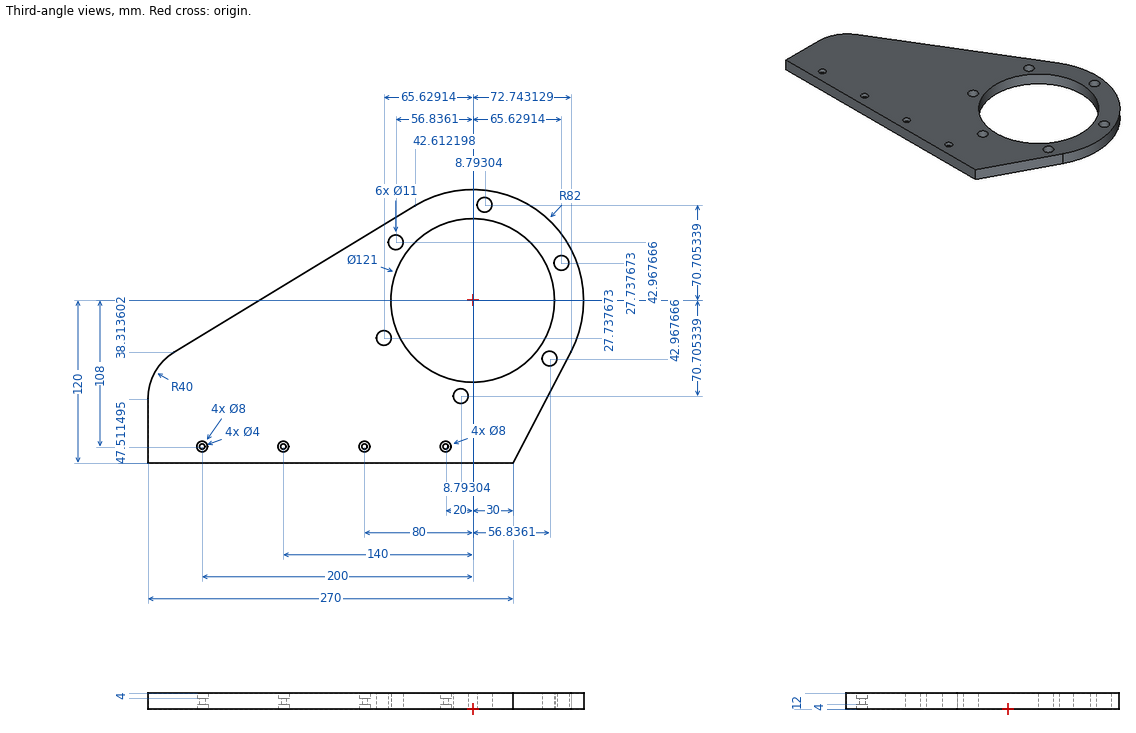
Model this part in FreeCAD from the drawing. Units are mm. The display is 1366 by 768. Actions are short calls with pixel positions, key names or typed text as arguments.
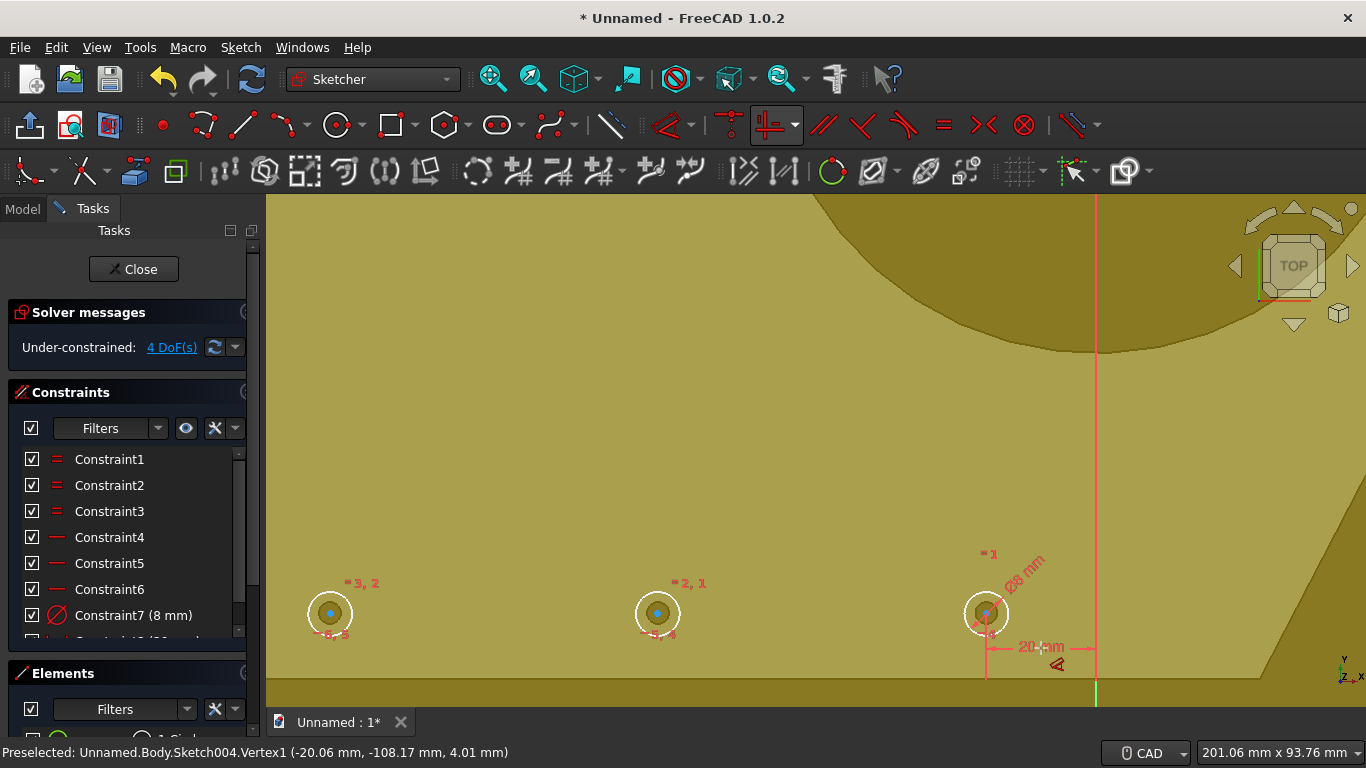
click(658, 614)
click(877, 648)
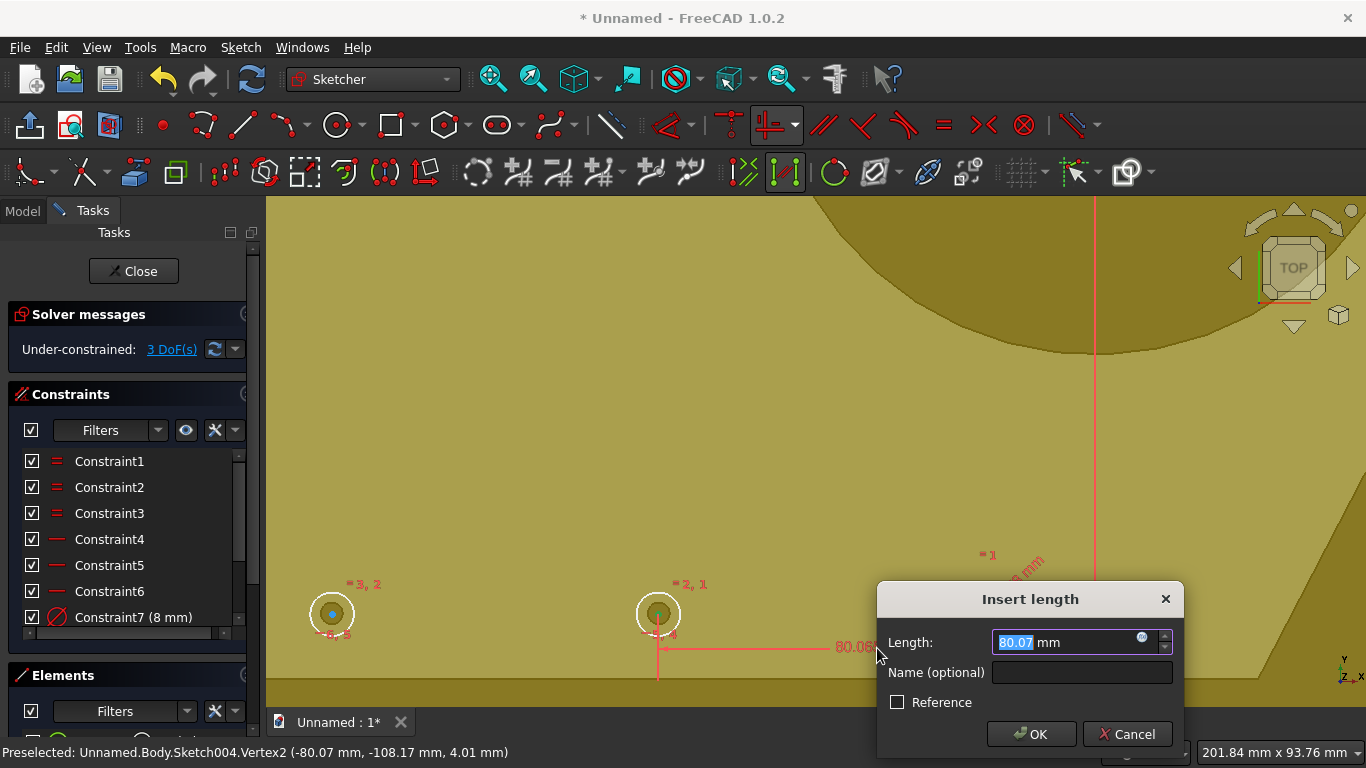
text(80)
key(Return)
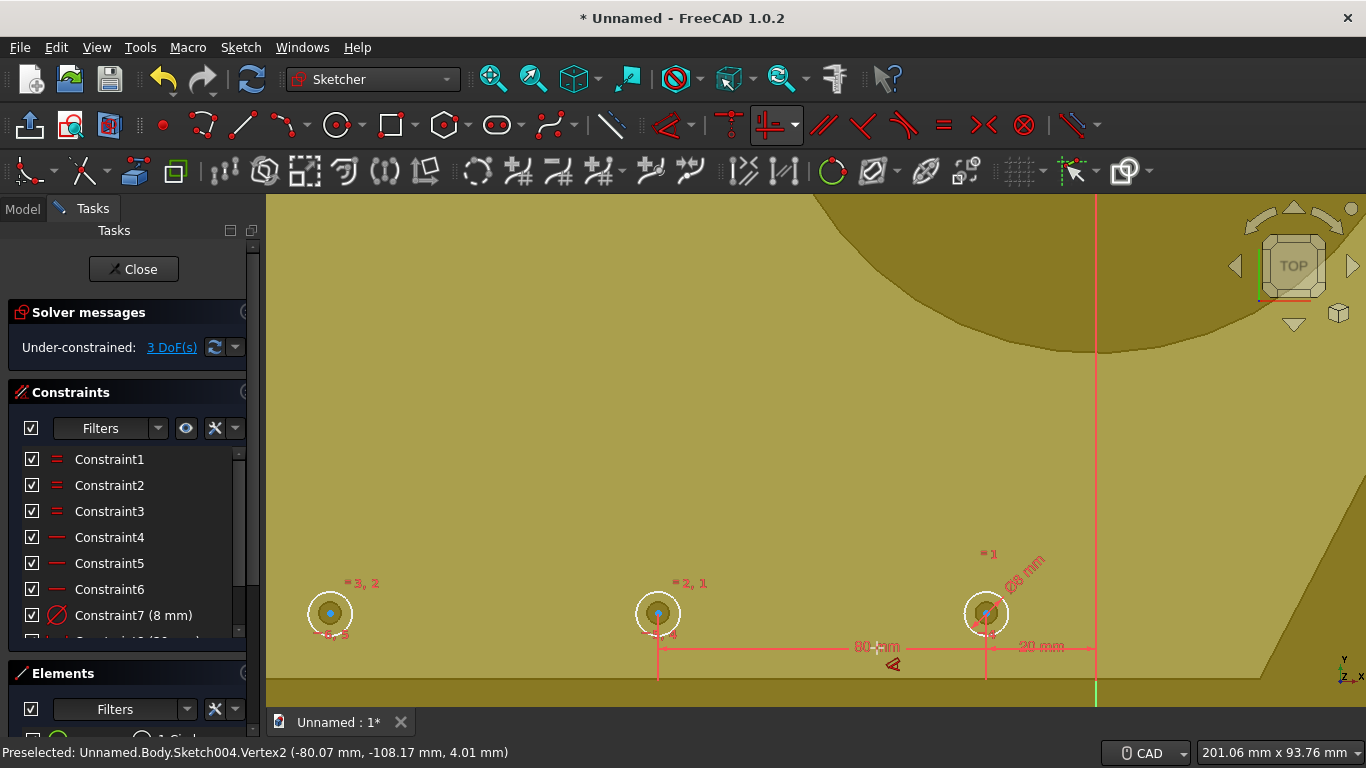
click(986, 614)
click(1130, 418)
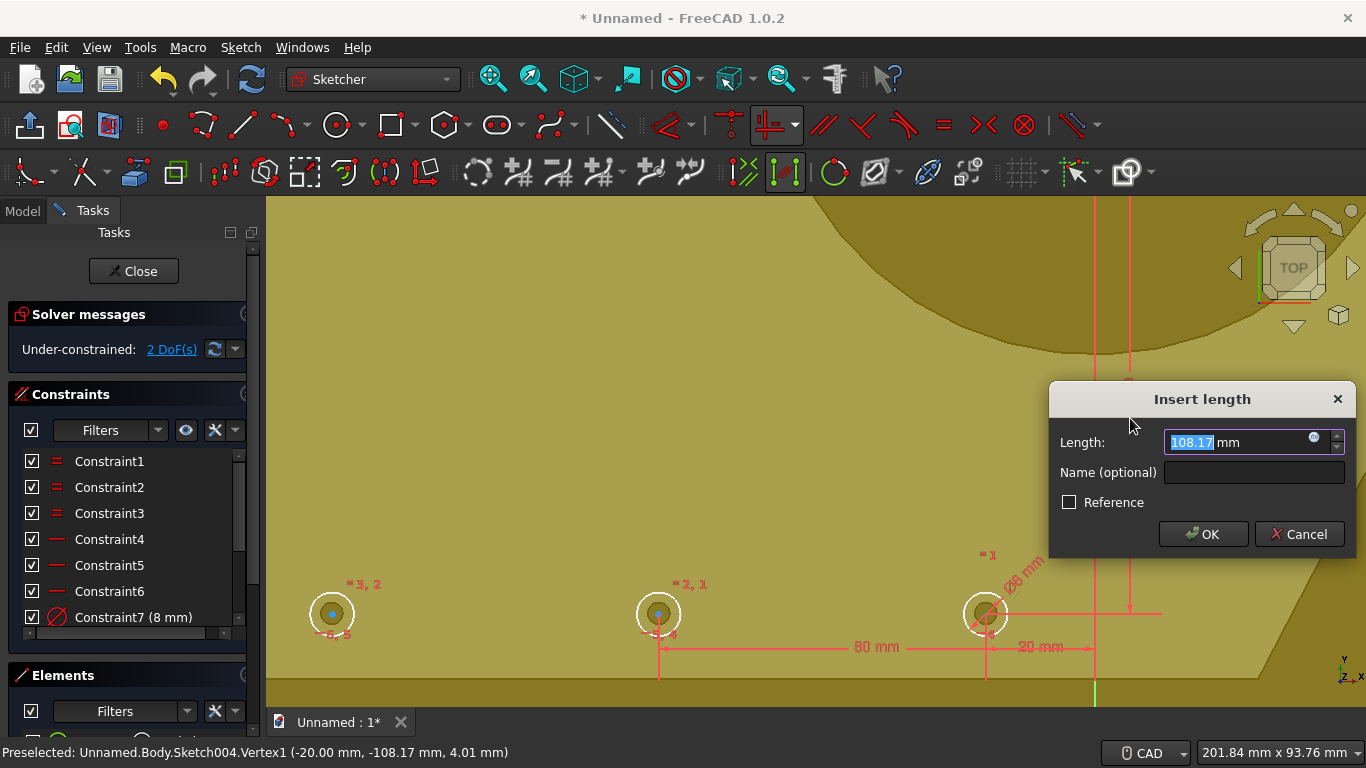
text(108)
key(Return)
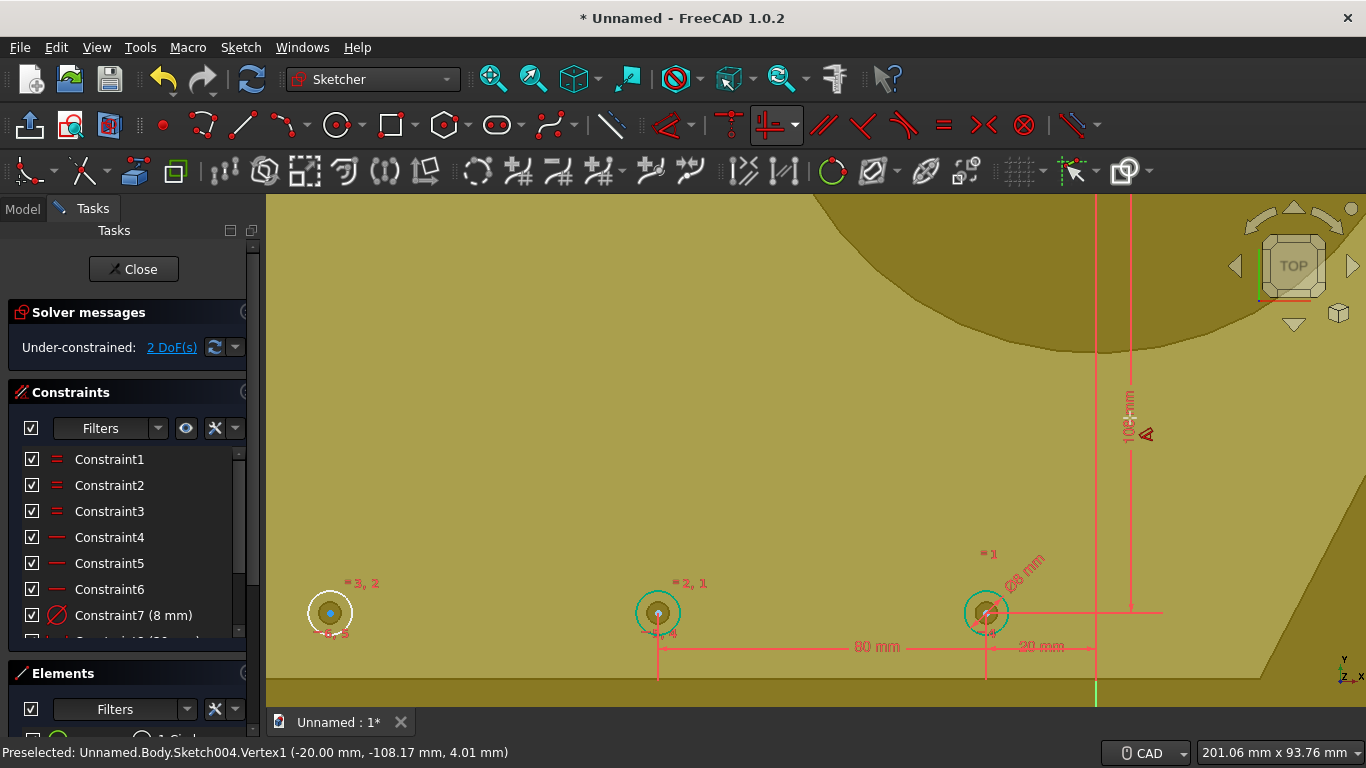
click(330, 613)
click(713, 647)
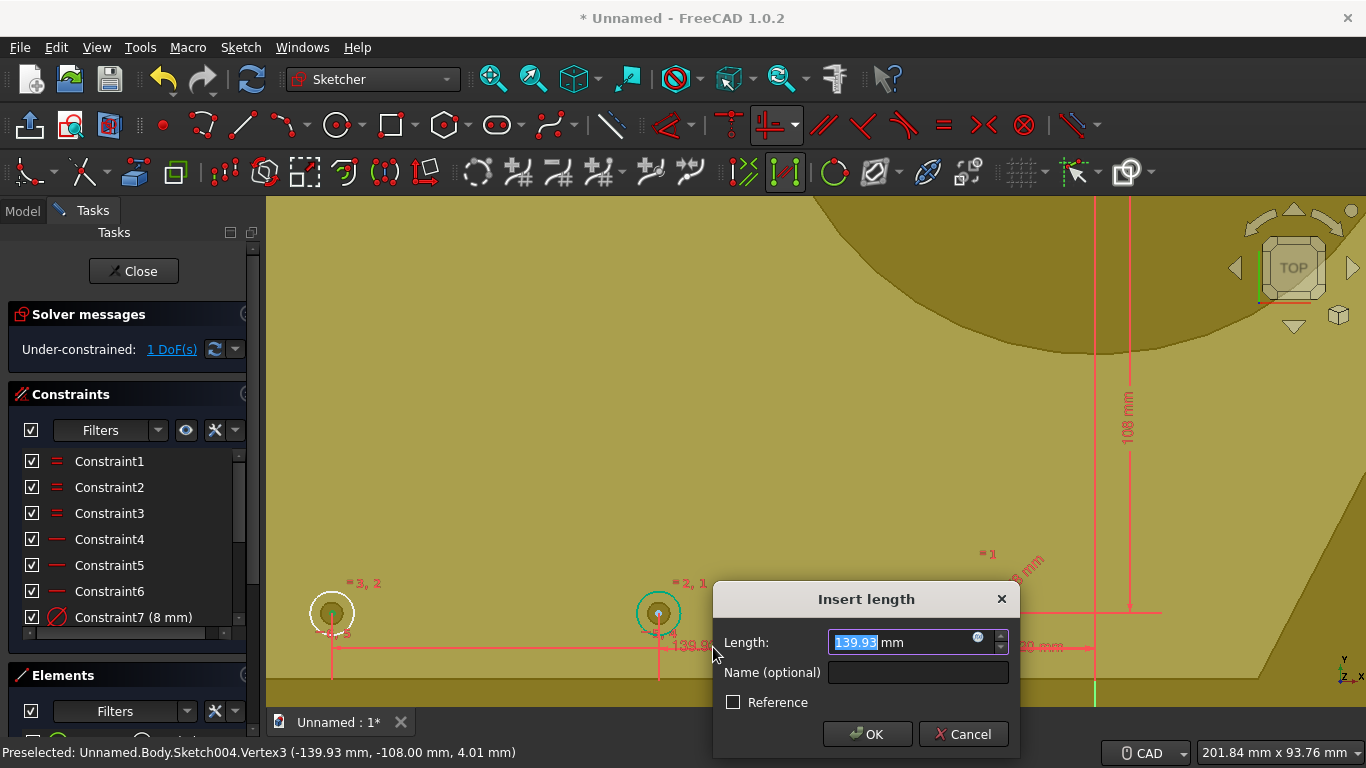
text(140)
key(Return)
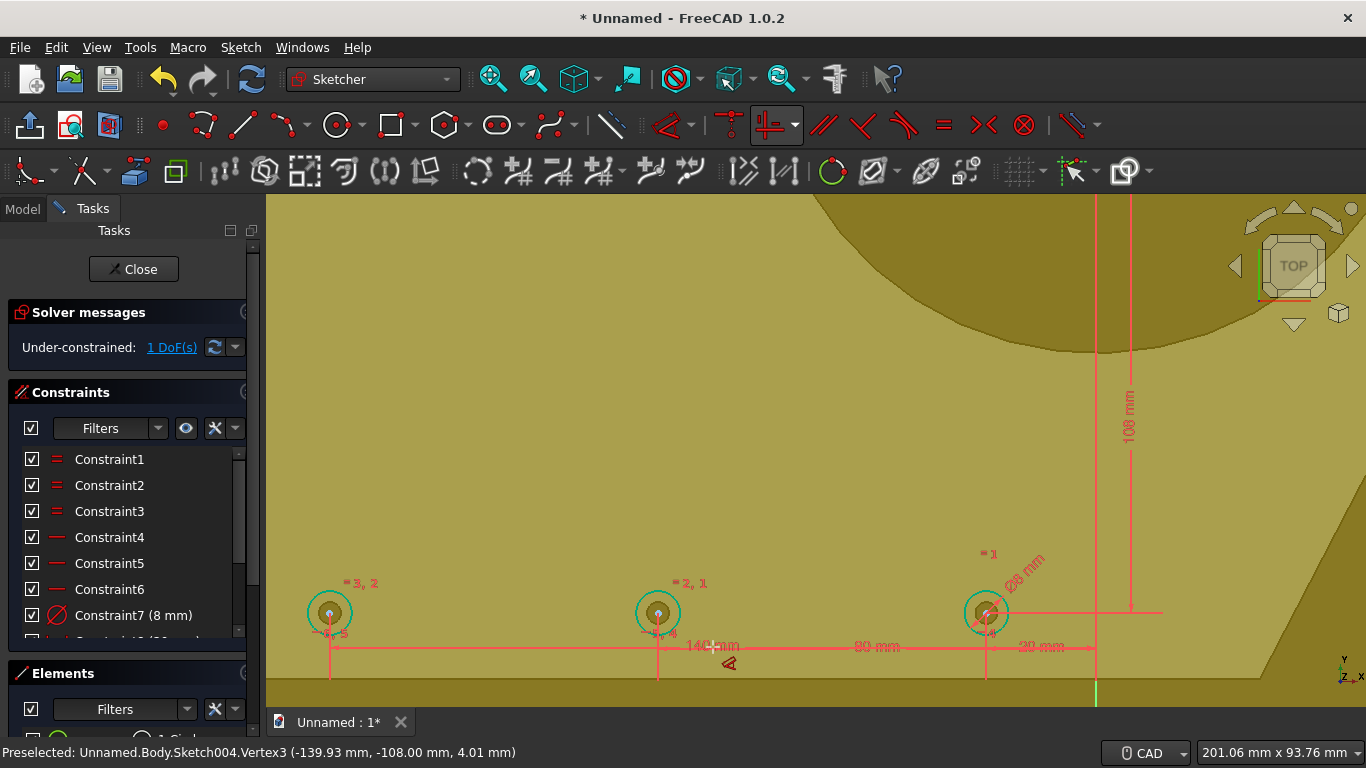
scroll(1003, 599, down, 3)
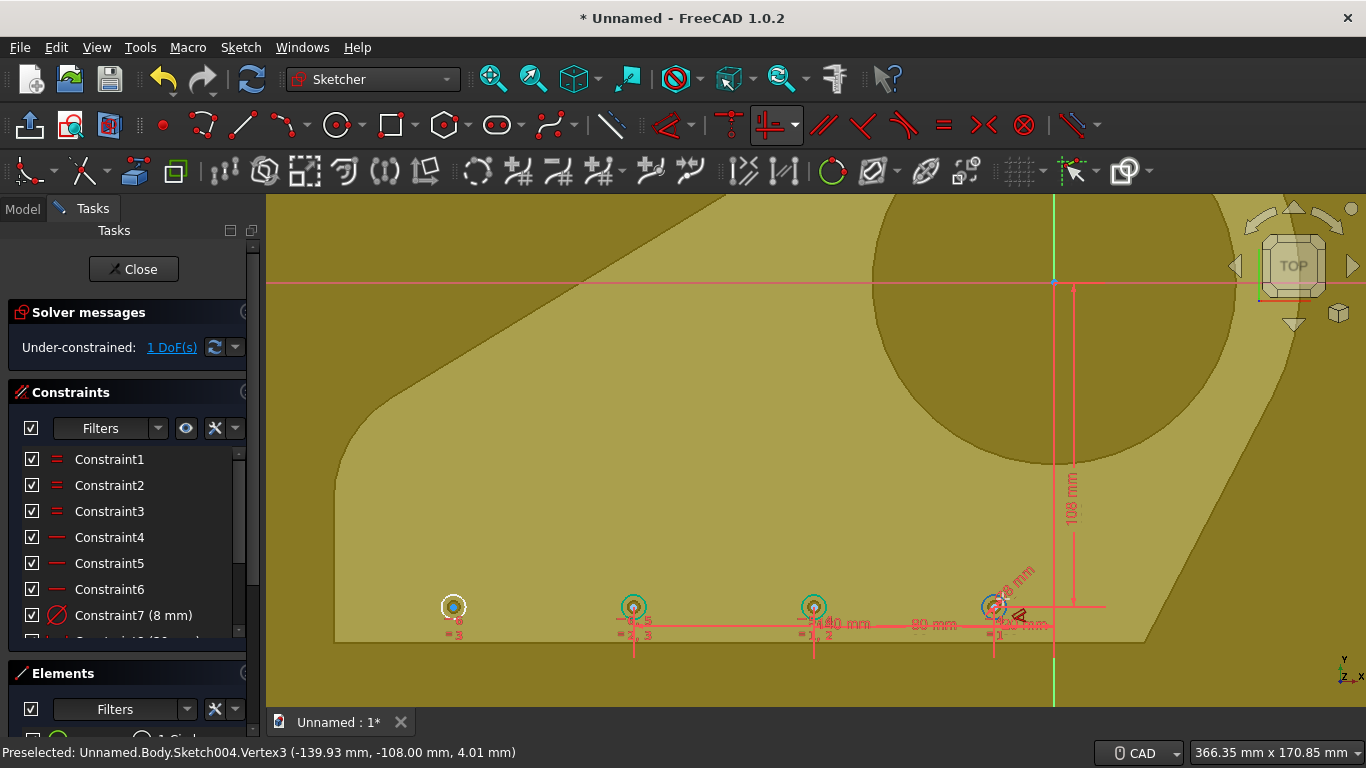
click(454, 607)
click(754, 249)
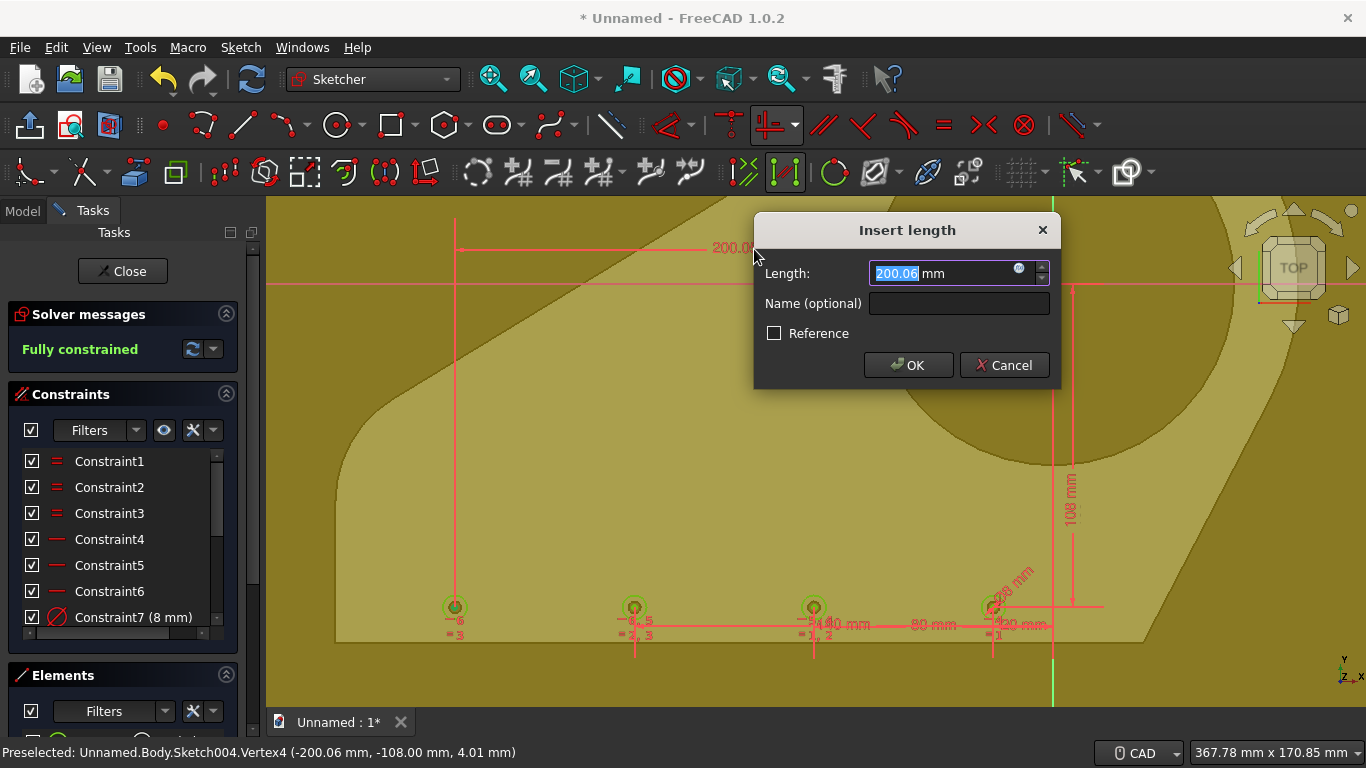
text(200)
key(Return)
key(Escape)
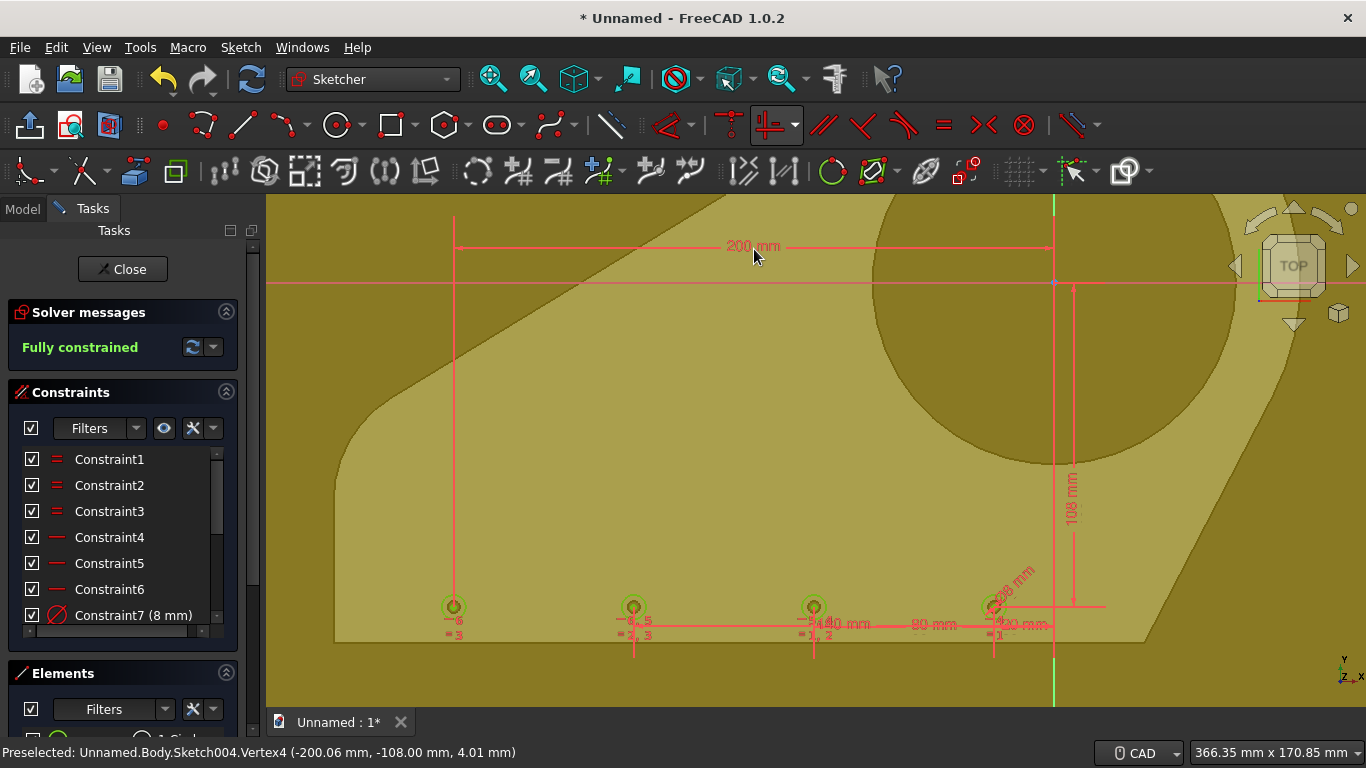
click(123, 269)